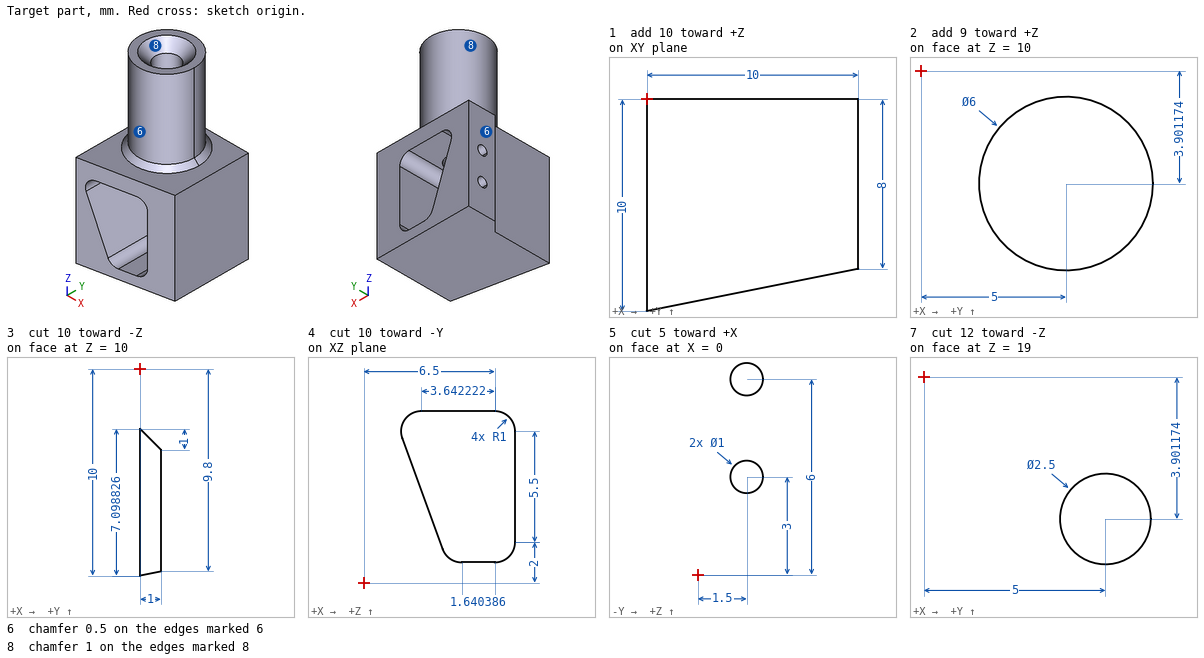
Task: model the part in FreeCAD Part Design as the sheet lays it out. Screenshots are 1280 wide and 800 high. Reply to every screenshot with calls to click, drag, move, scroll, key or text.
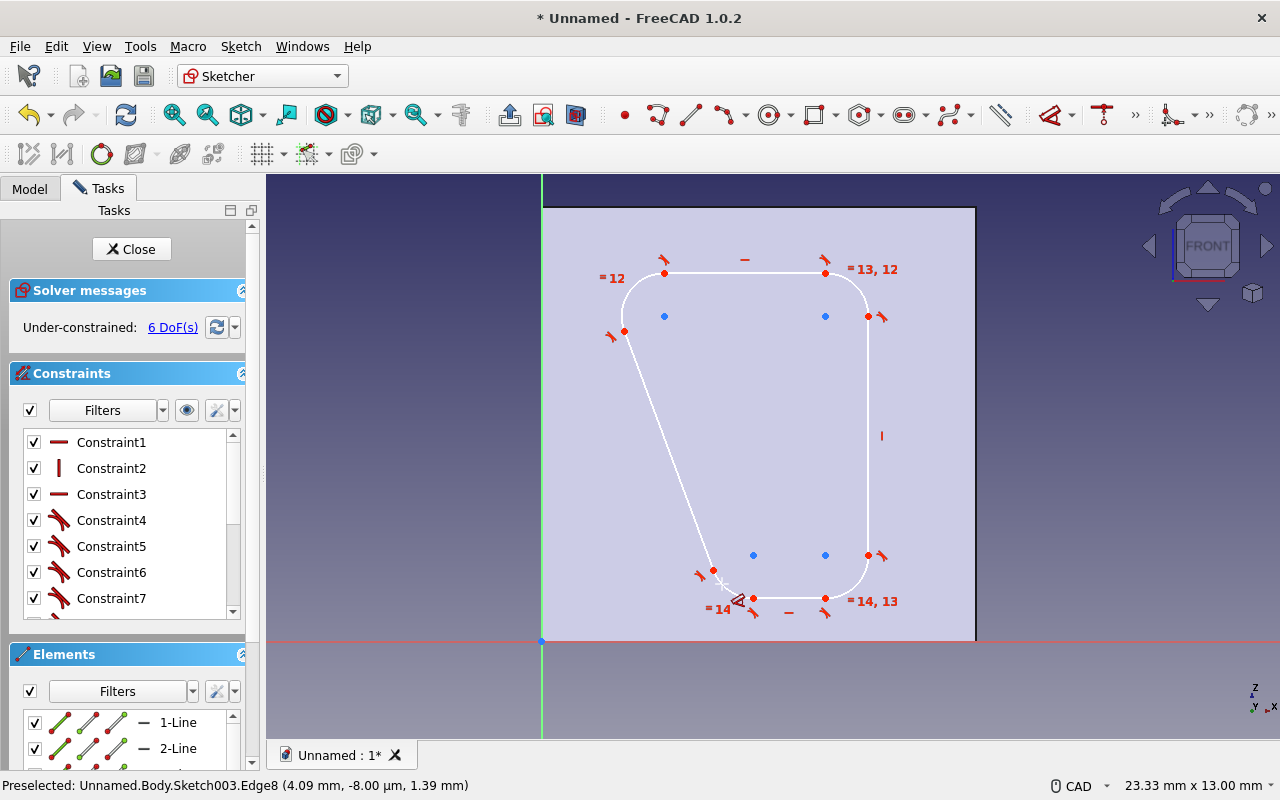
click(641, 280)
click(624, 253)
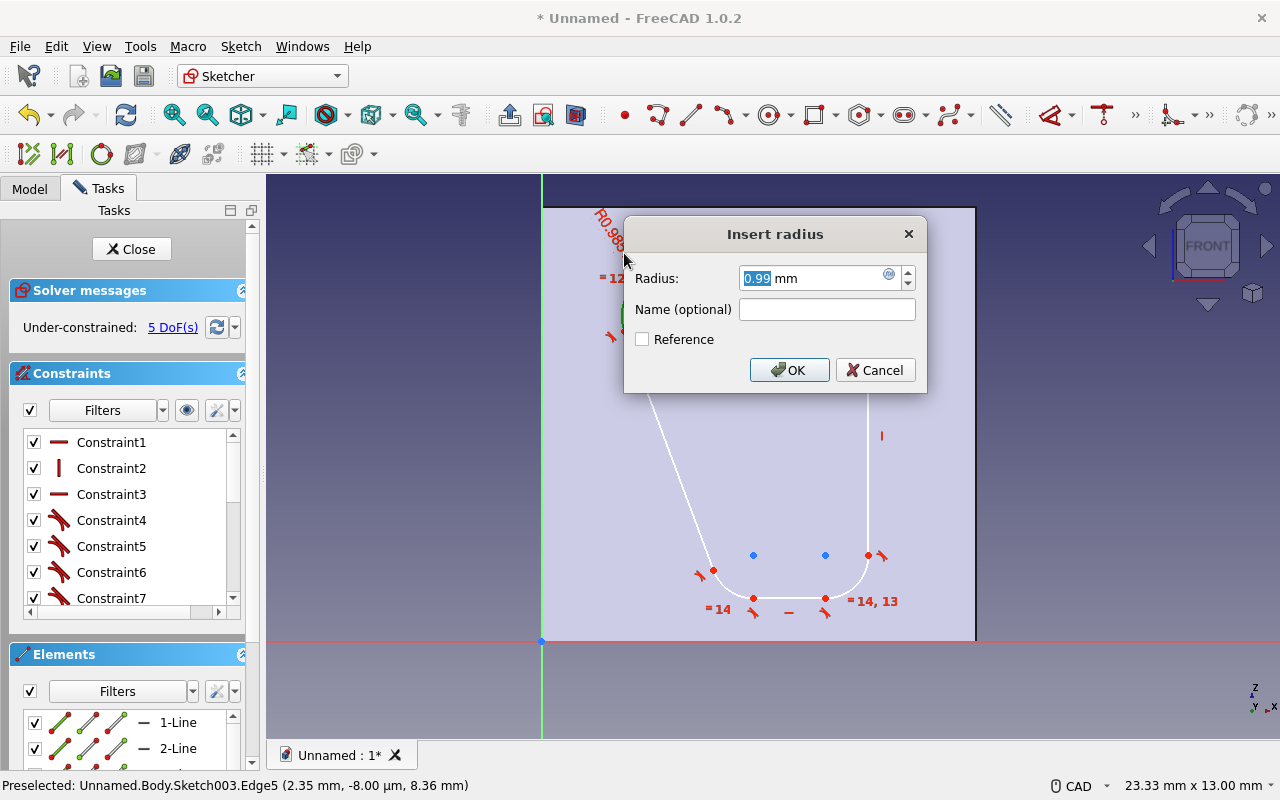
text(1)
key(Return)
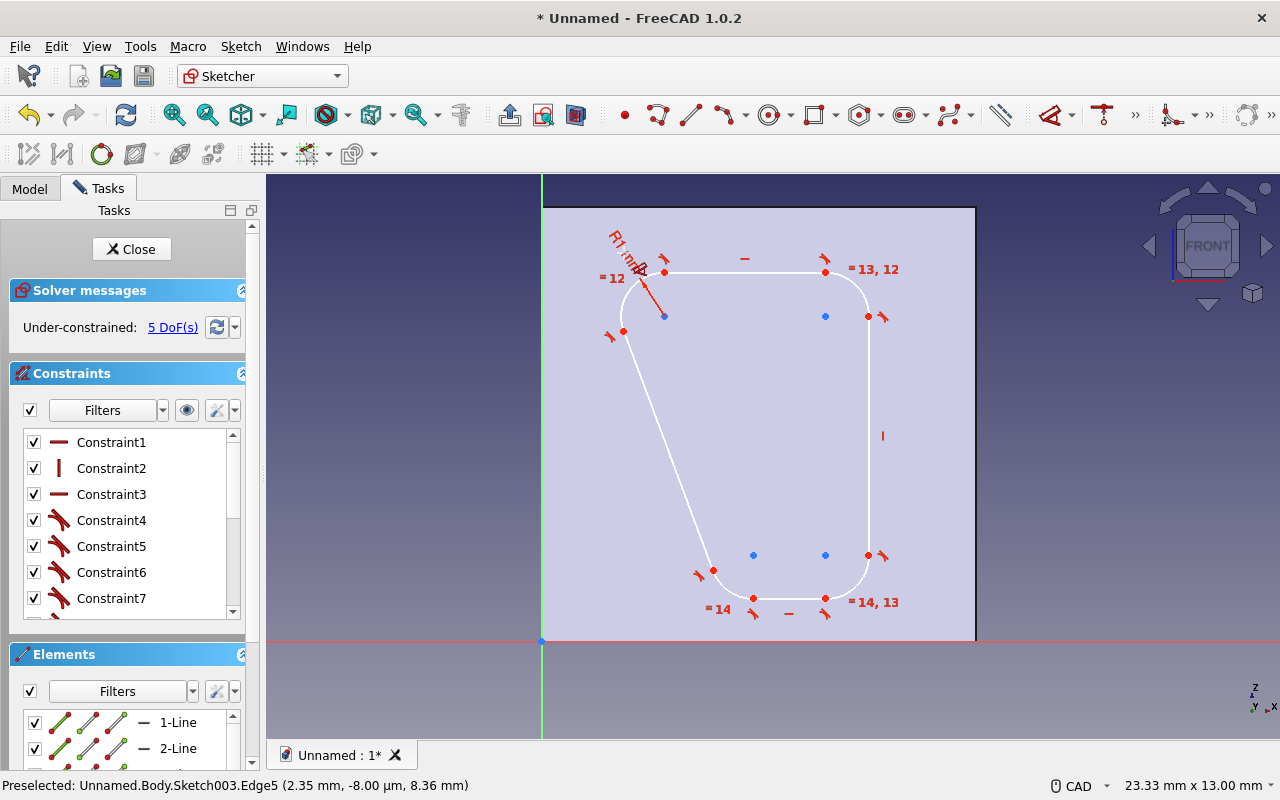
click(869, 555)
click(903, 599)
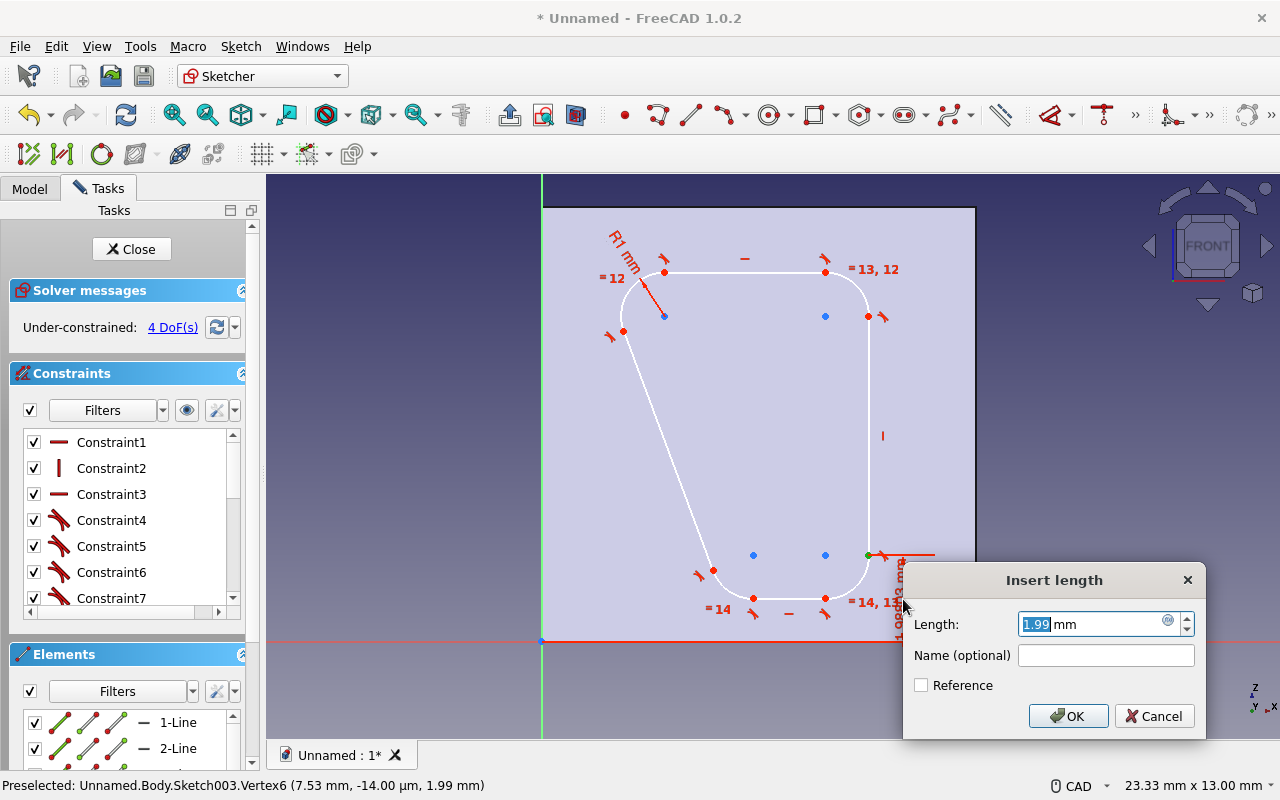
text(2)
key(Return)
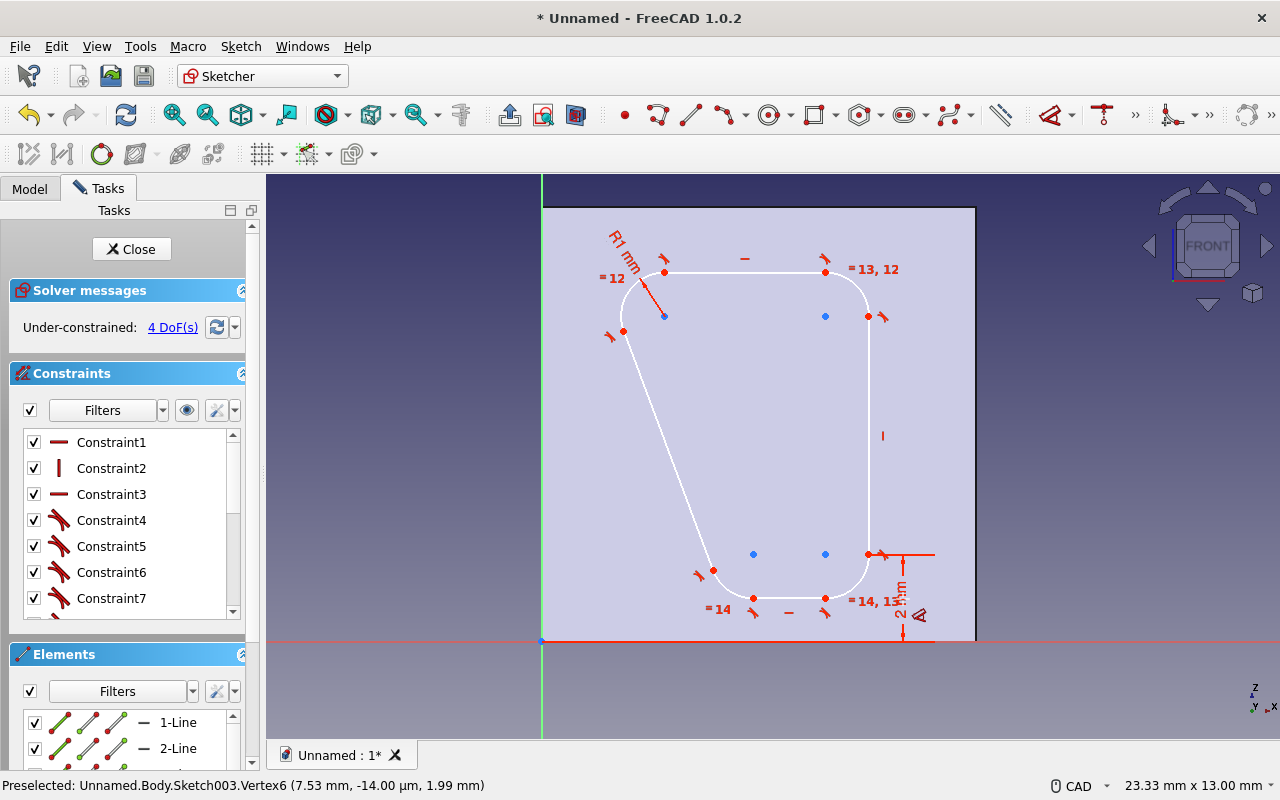
click(869, 388)
click(903, 436)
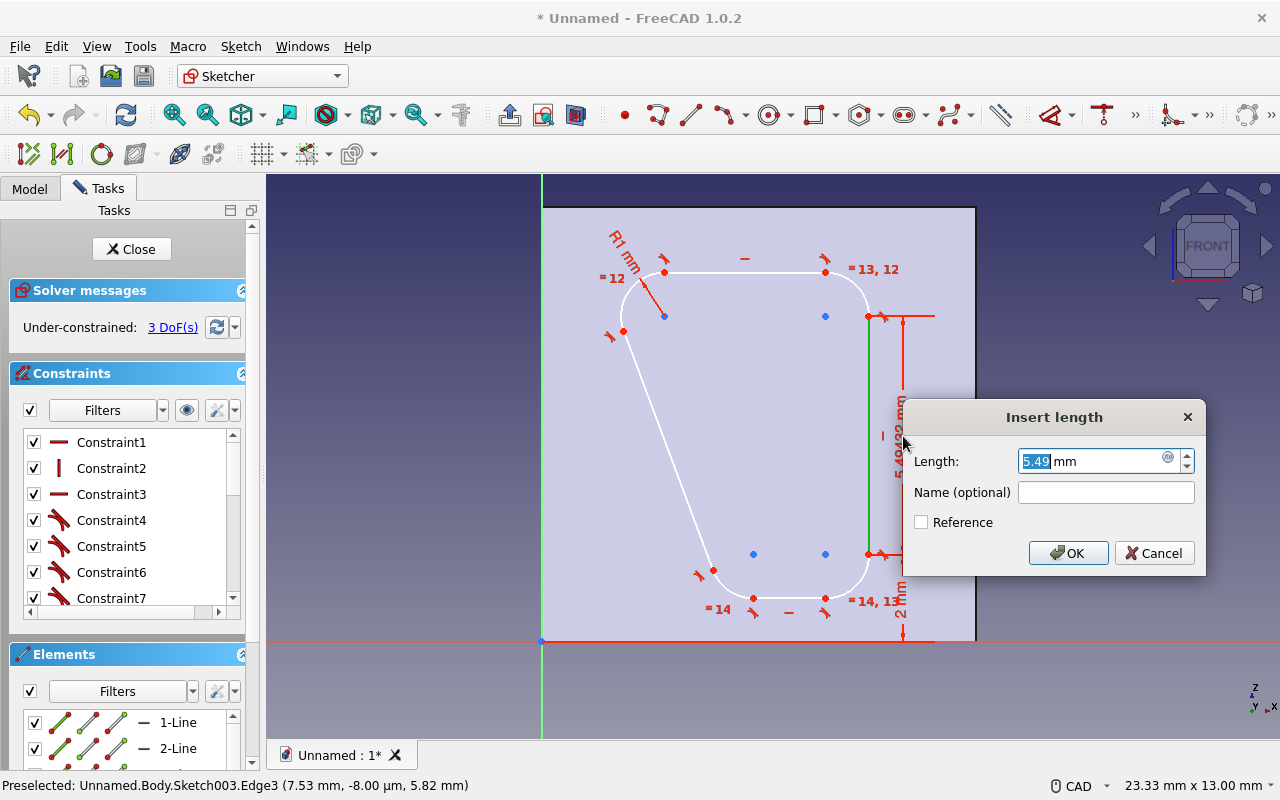
text(5.5)
key(Return)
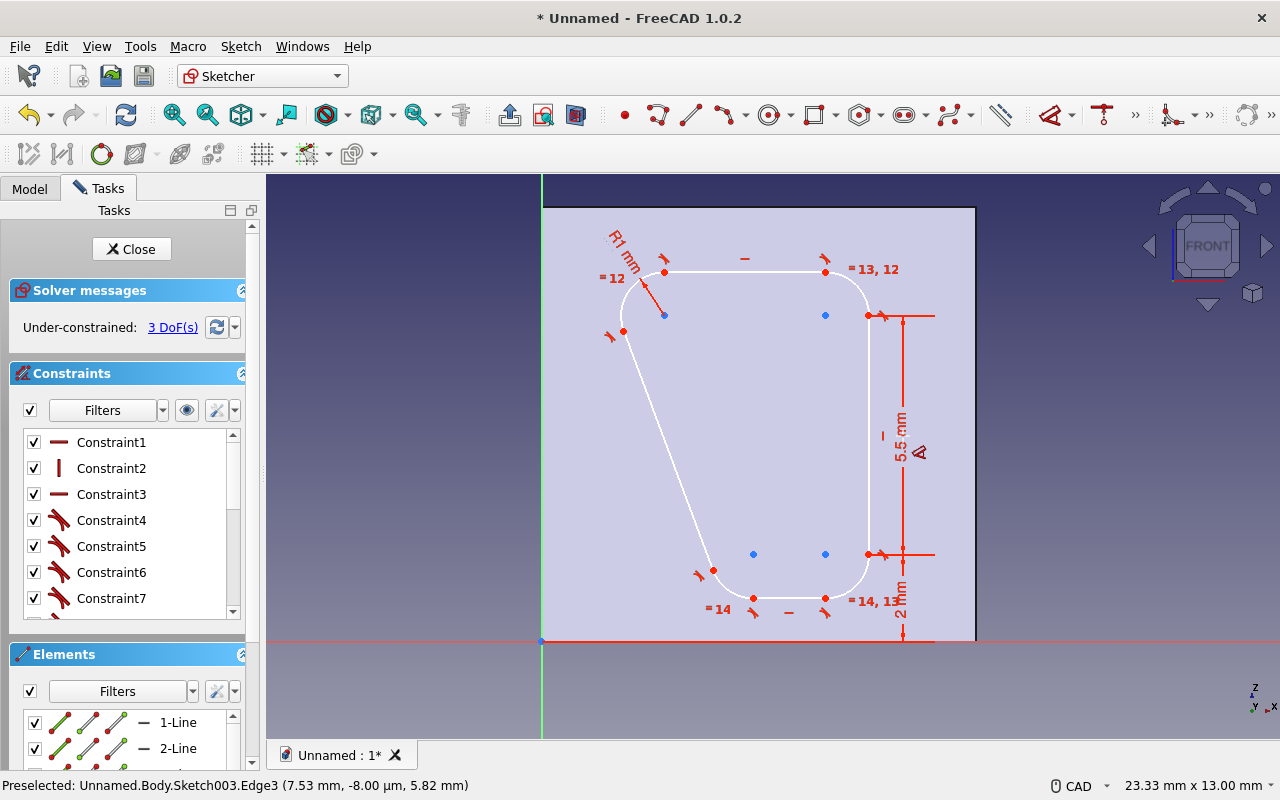
click(826, 272)
click(684, 676)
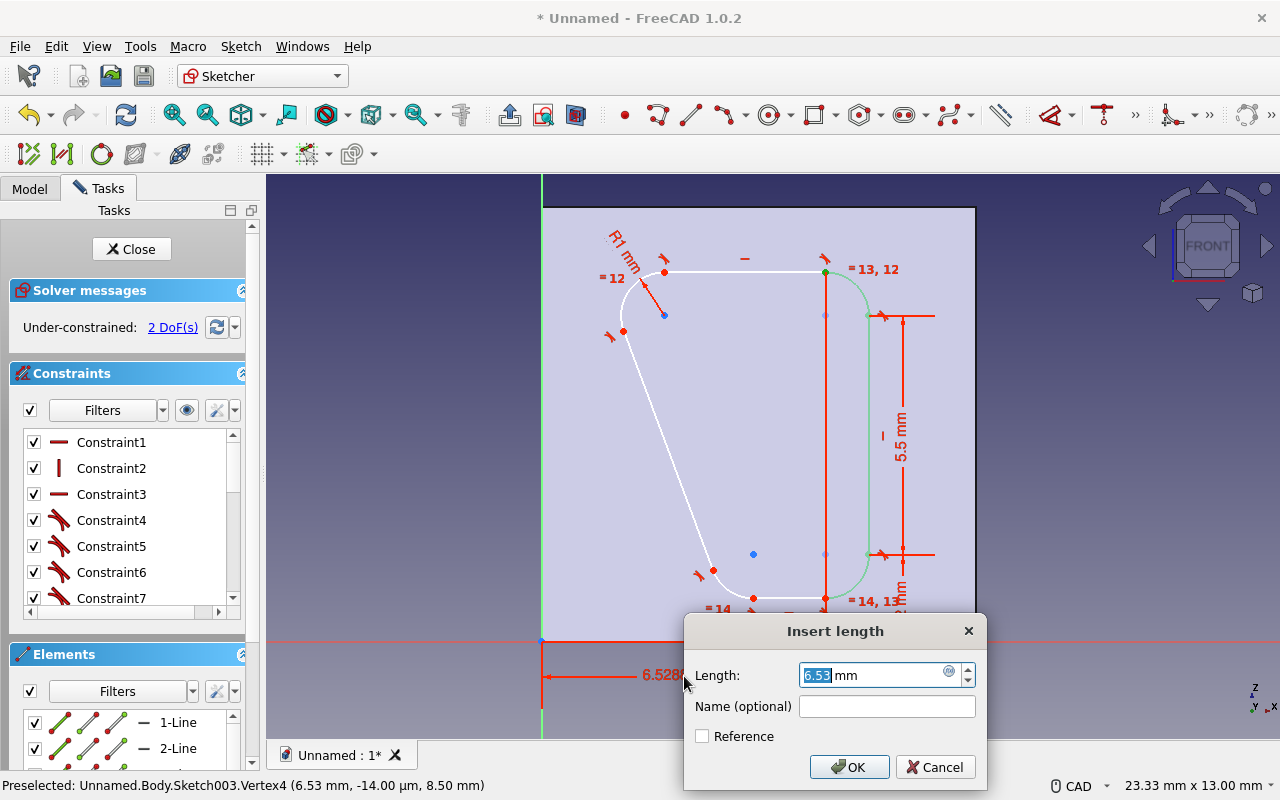
text(6.5)
key(Return)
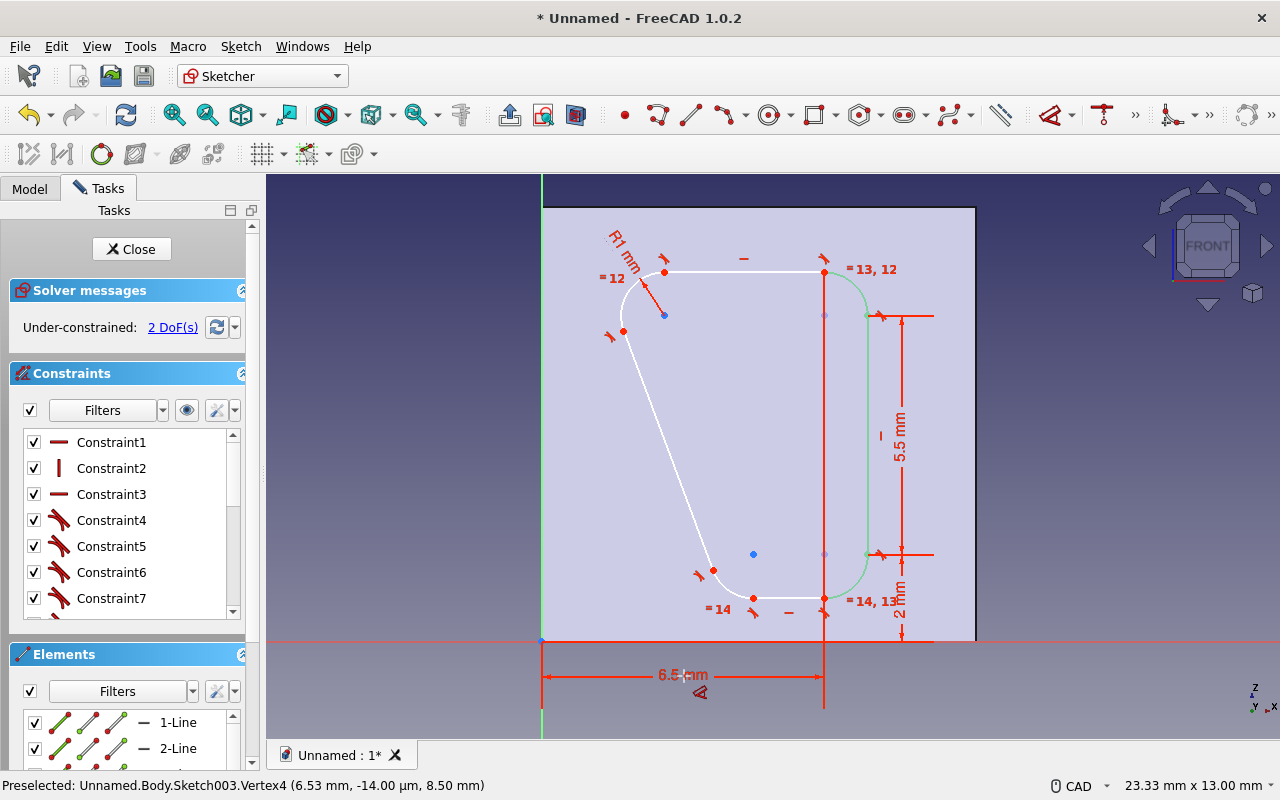
click(713, 272)
click(744, 238)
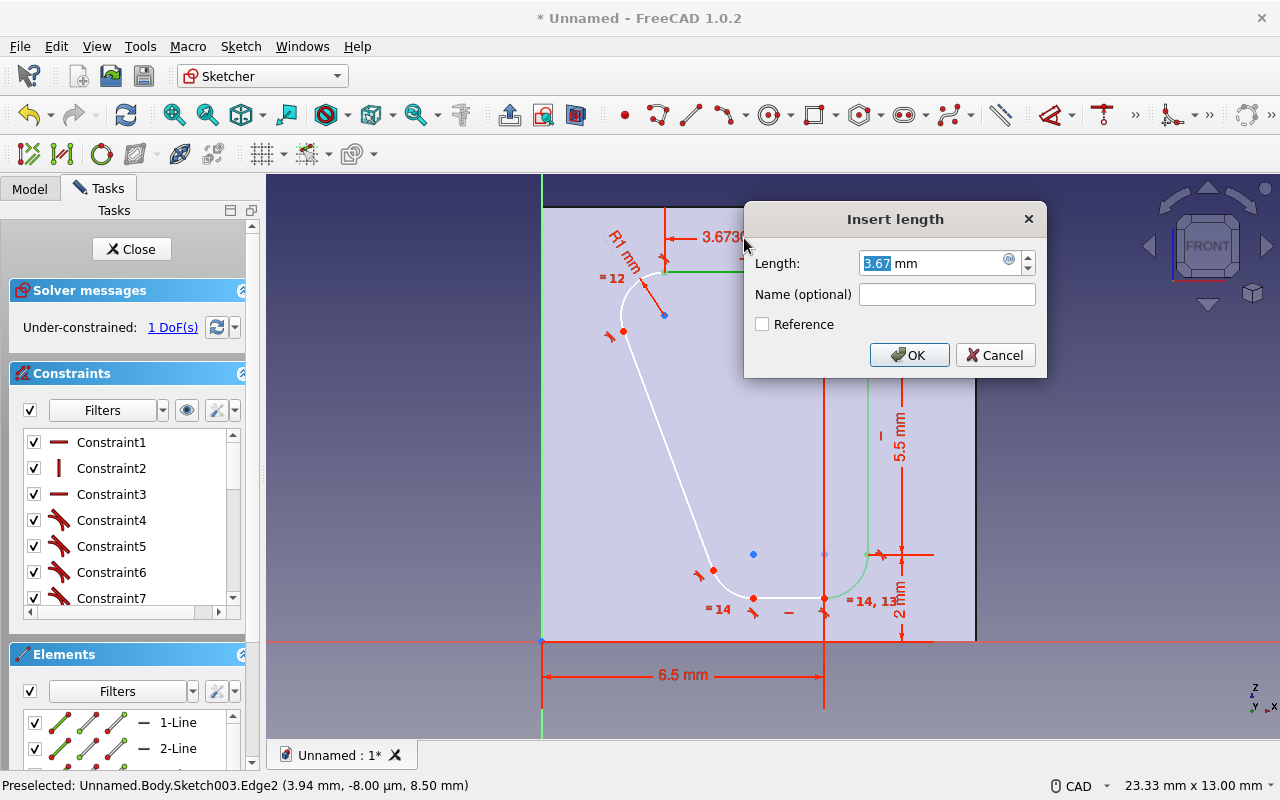
text(3.642222)
key(Return)